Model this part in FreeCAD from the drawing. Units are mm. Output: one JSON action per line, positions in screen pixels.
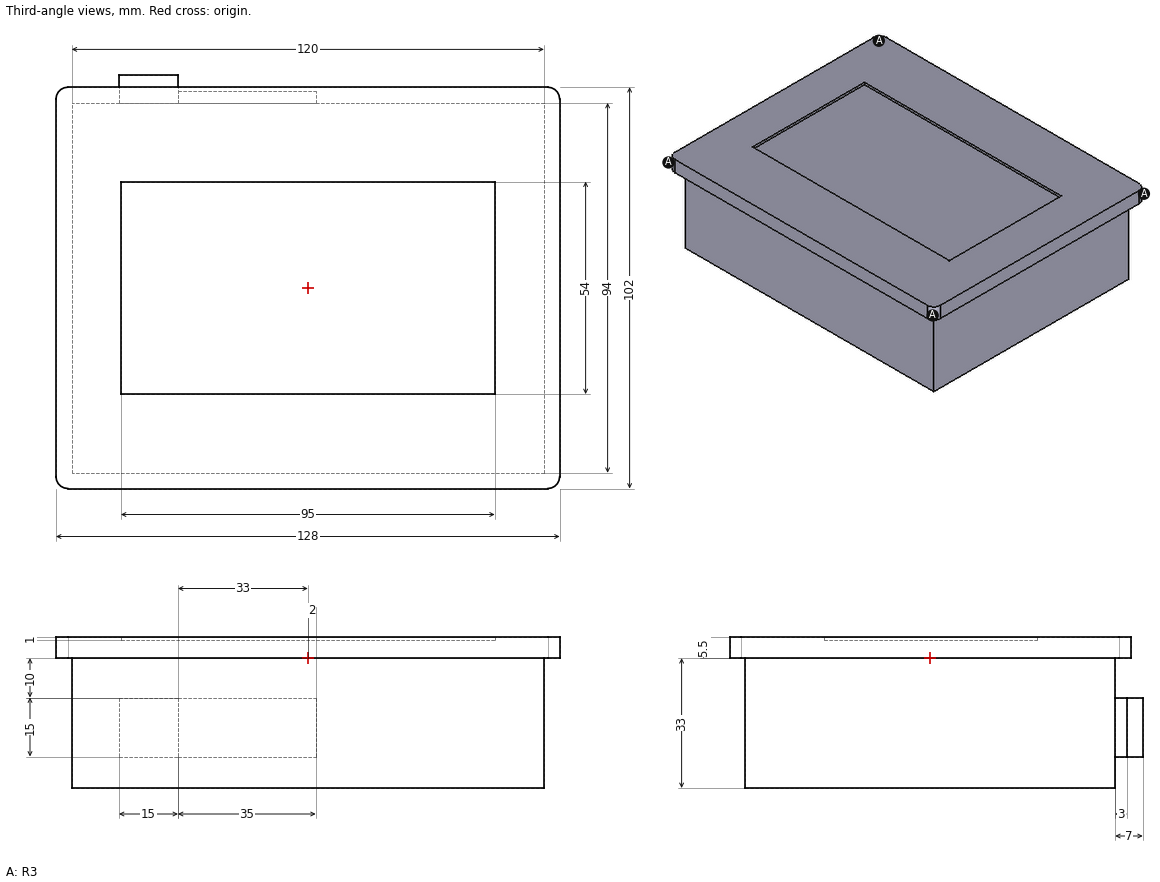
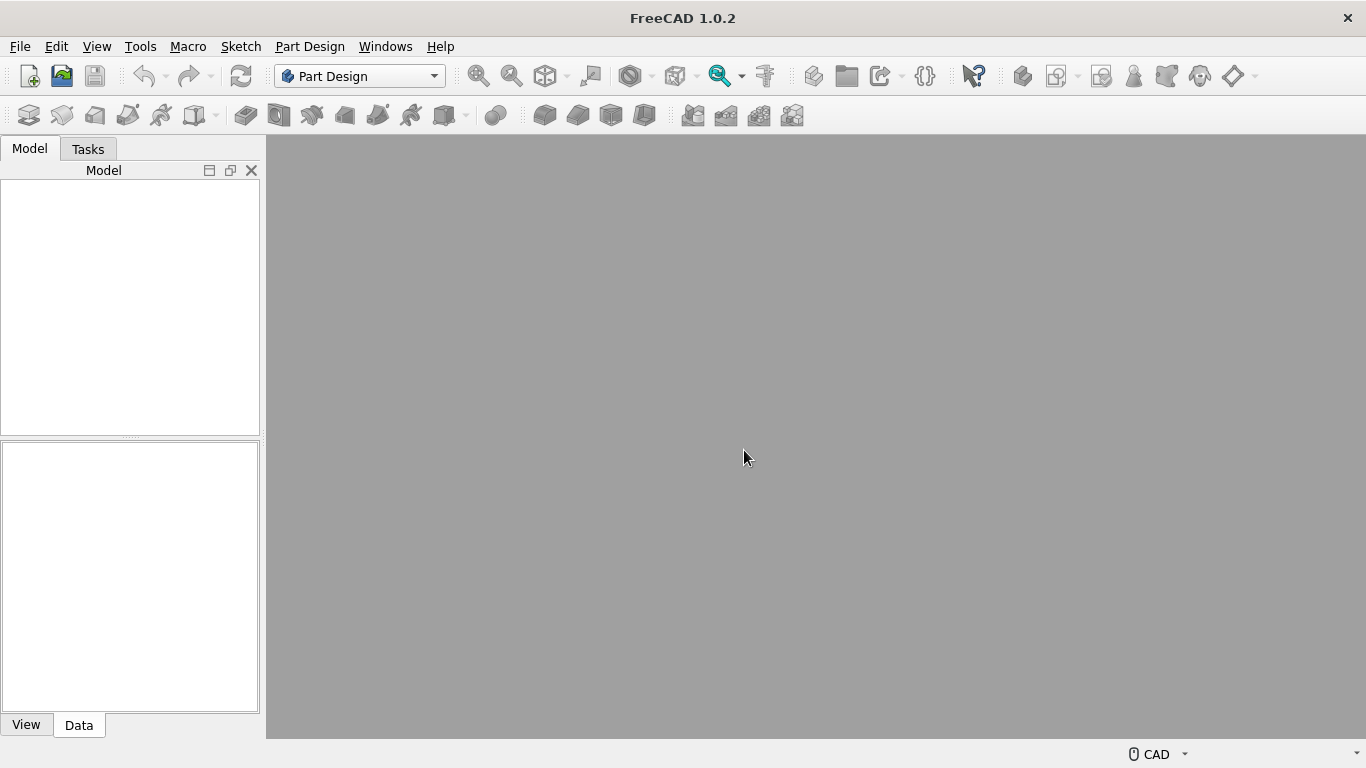
{"action": "key", "text": "ctrl+n"}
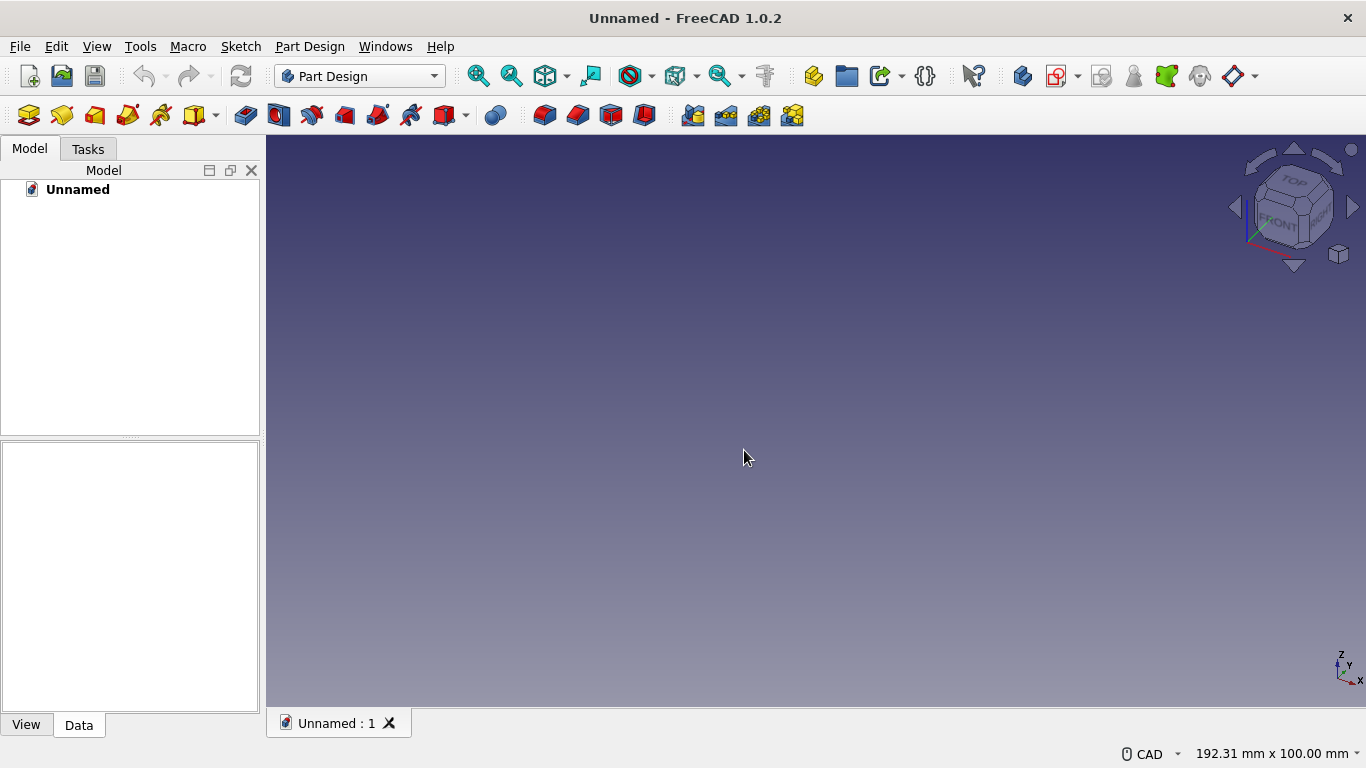
{"action": "left_click", "coordinate": [1056, 76]}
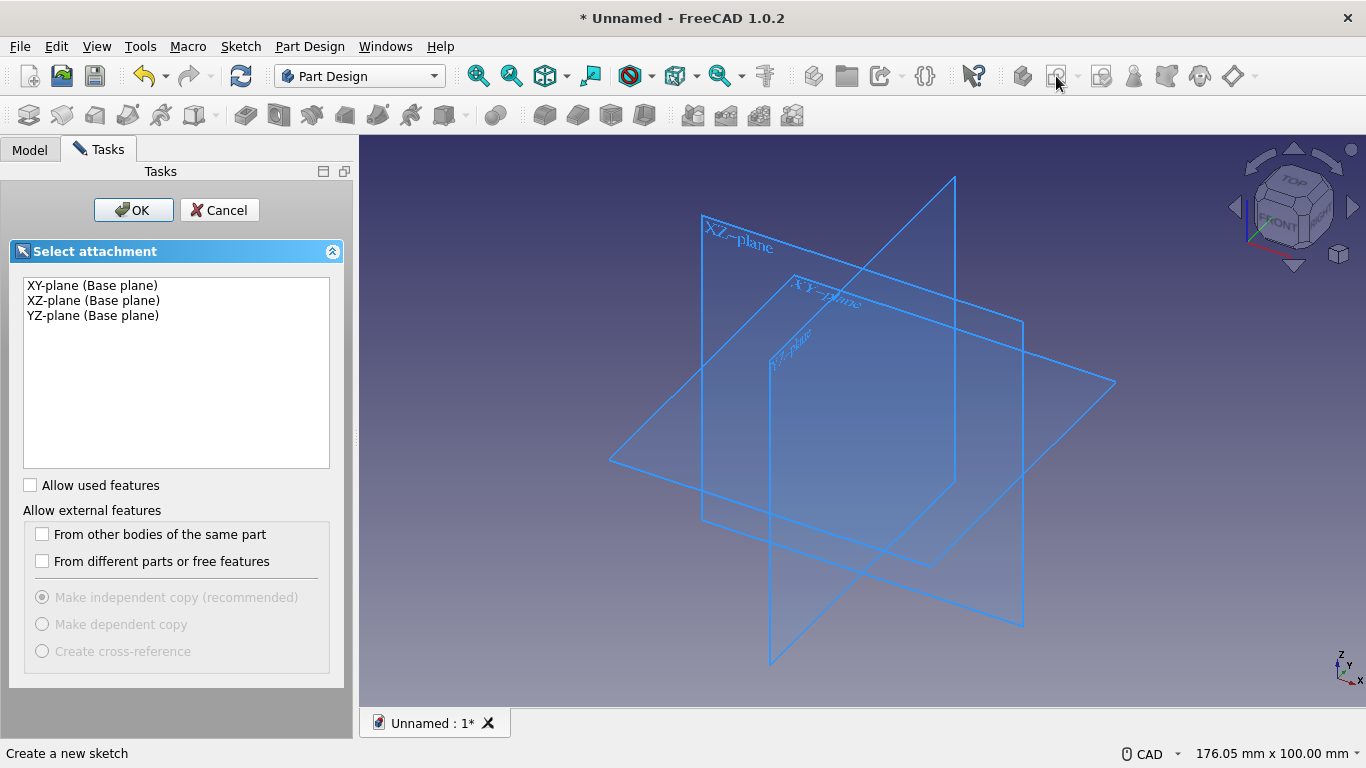
{"action": "left_click", "coordinate": [84, 286]}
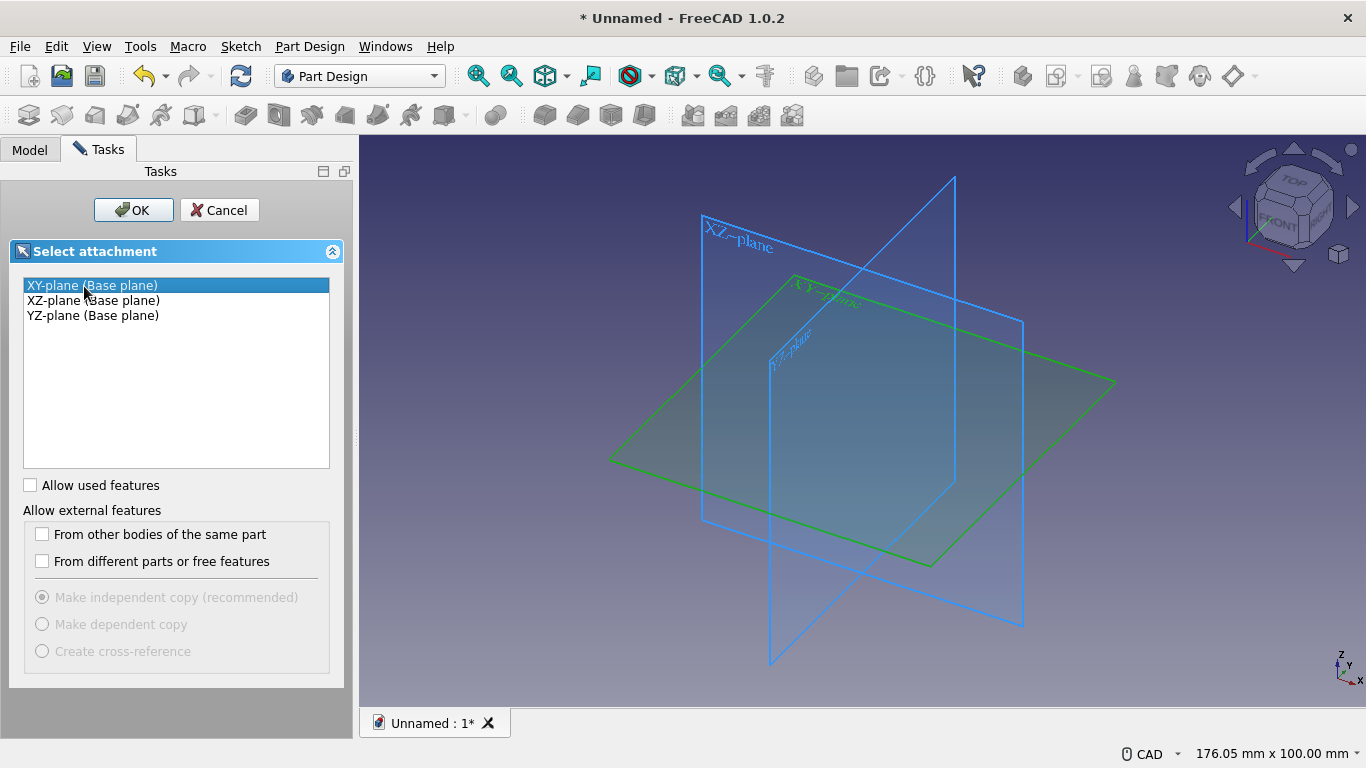
{"action": "left_click", "coordinate": [134, 210]}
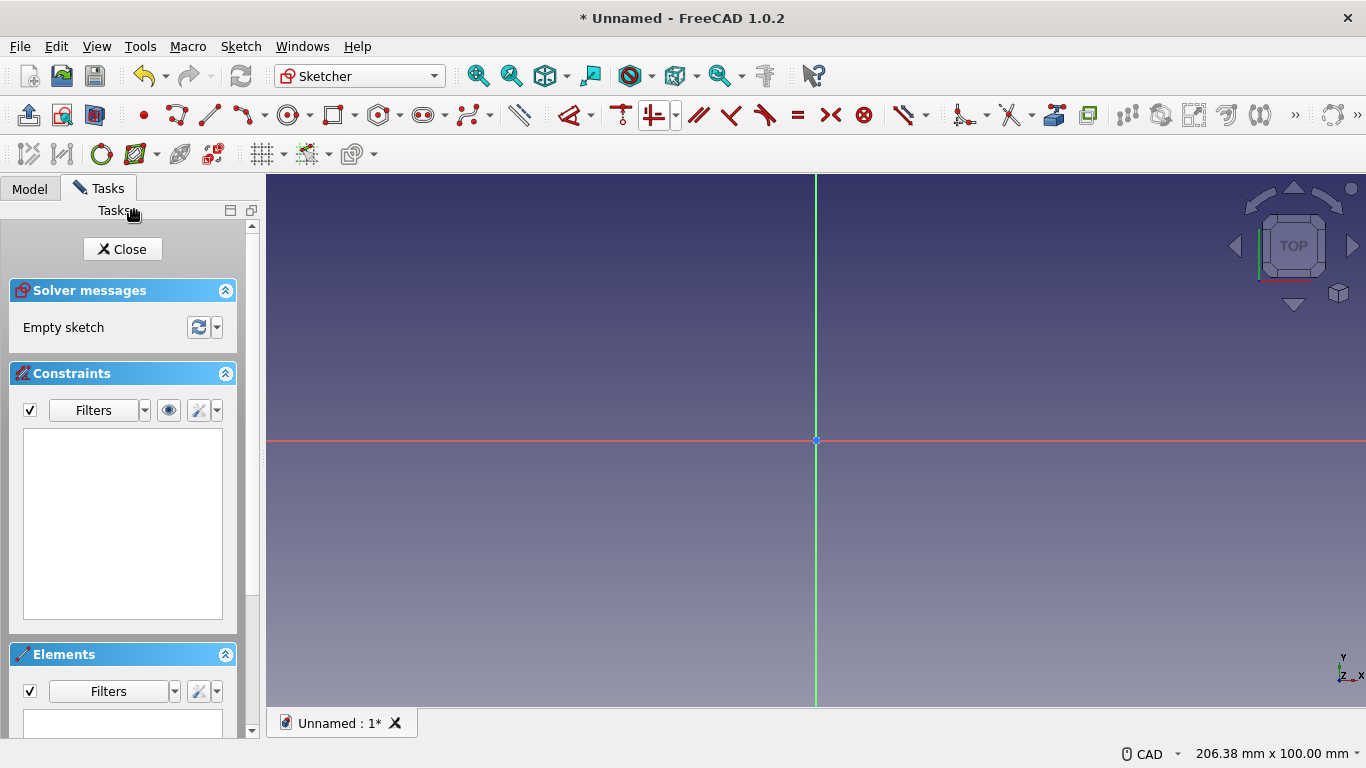
{"action": "scroll", "coordinate": [608, 440], "scroll_direction": "down", "scroll_amount": 2}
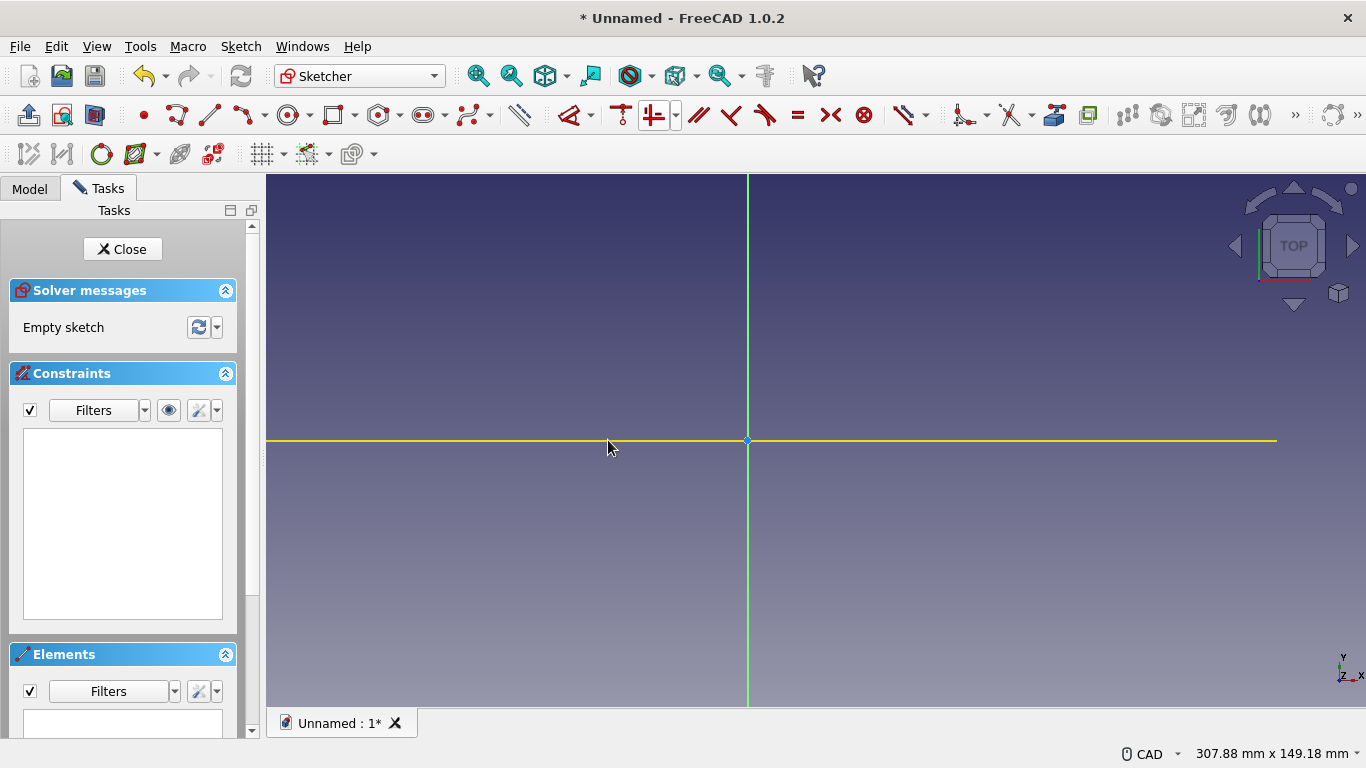
{"action": "left_click", "coordinate": [354, 116]}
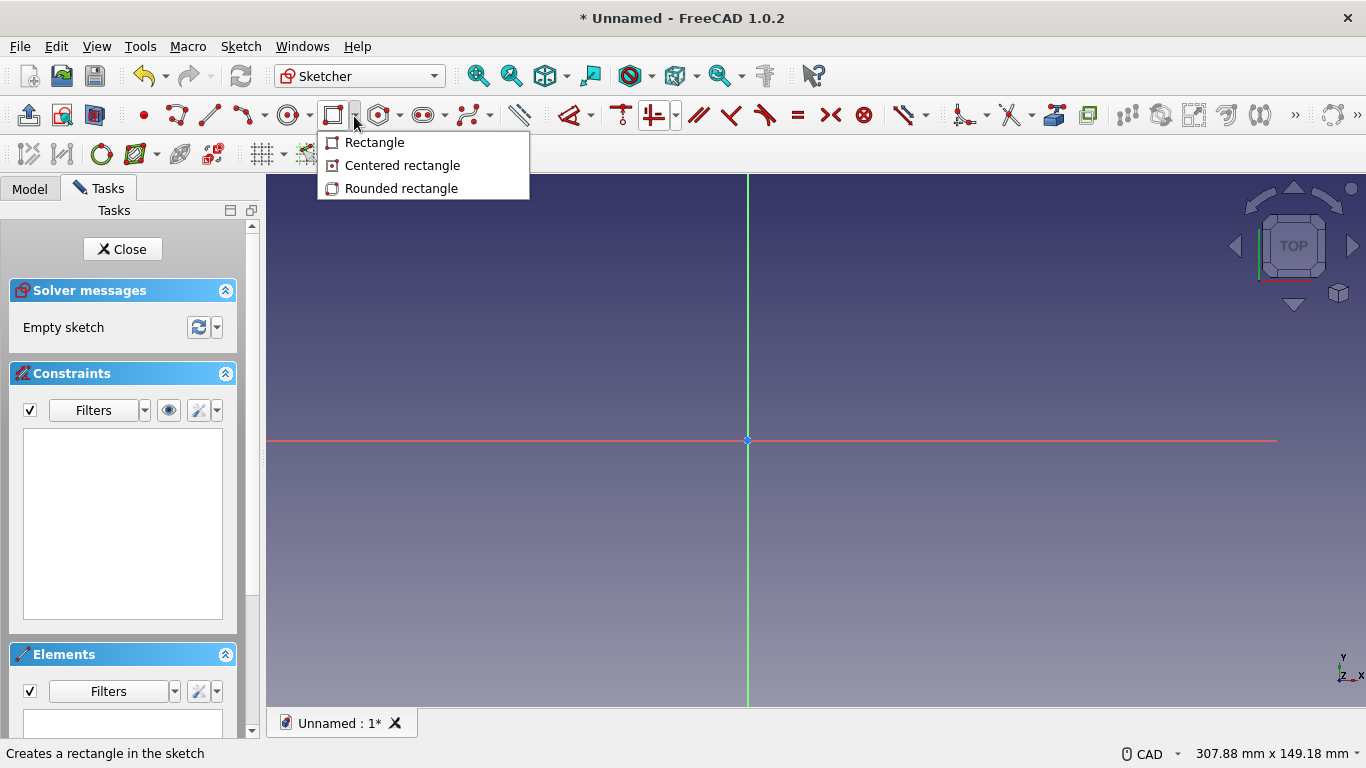
{"action": "left_click", "coordinate": [424, 166]}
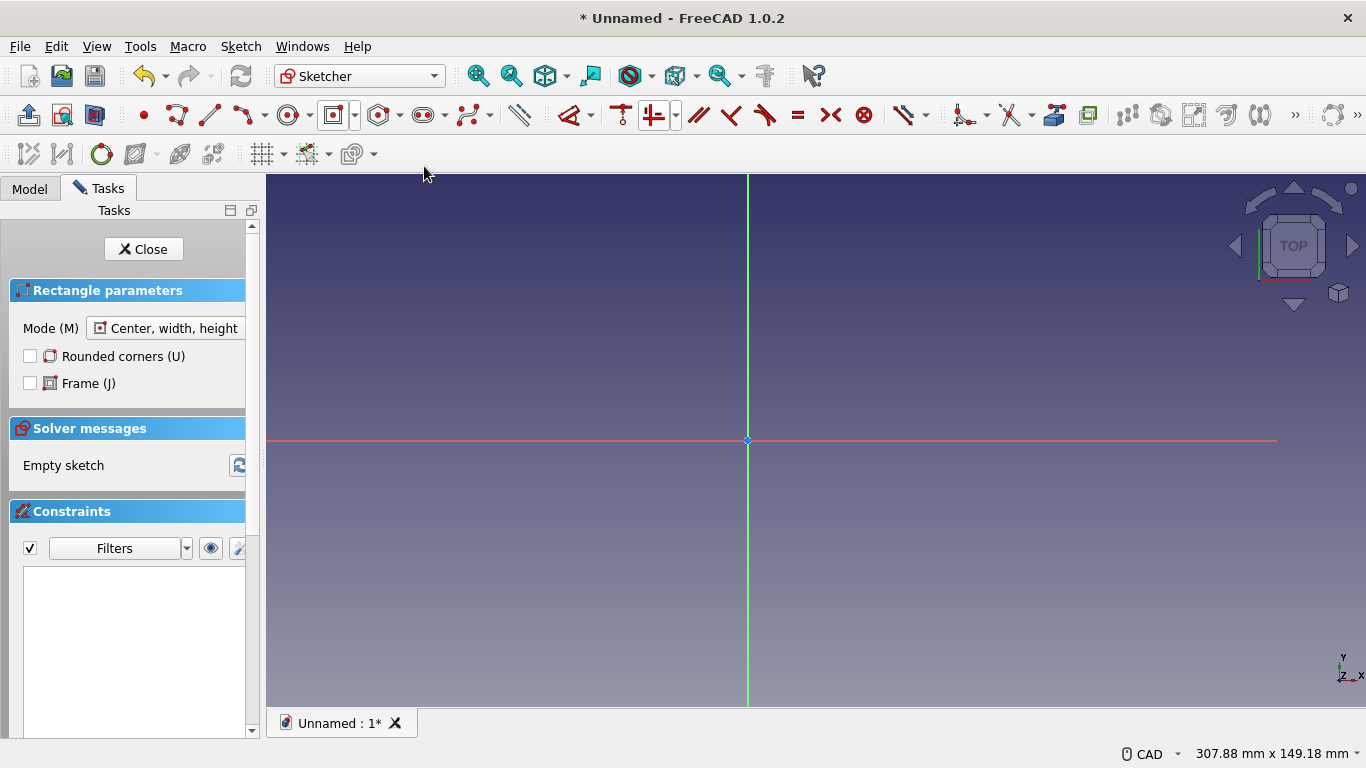
{"action": "left_click", "coordinate": [748, 440]}
{"action": "mouse_move", "coordinate": [976, 258]}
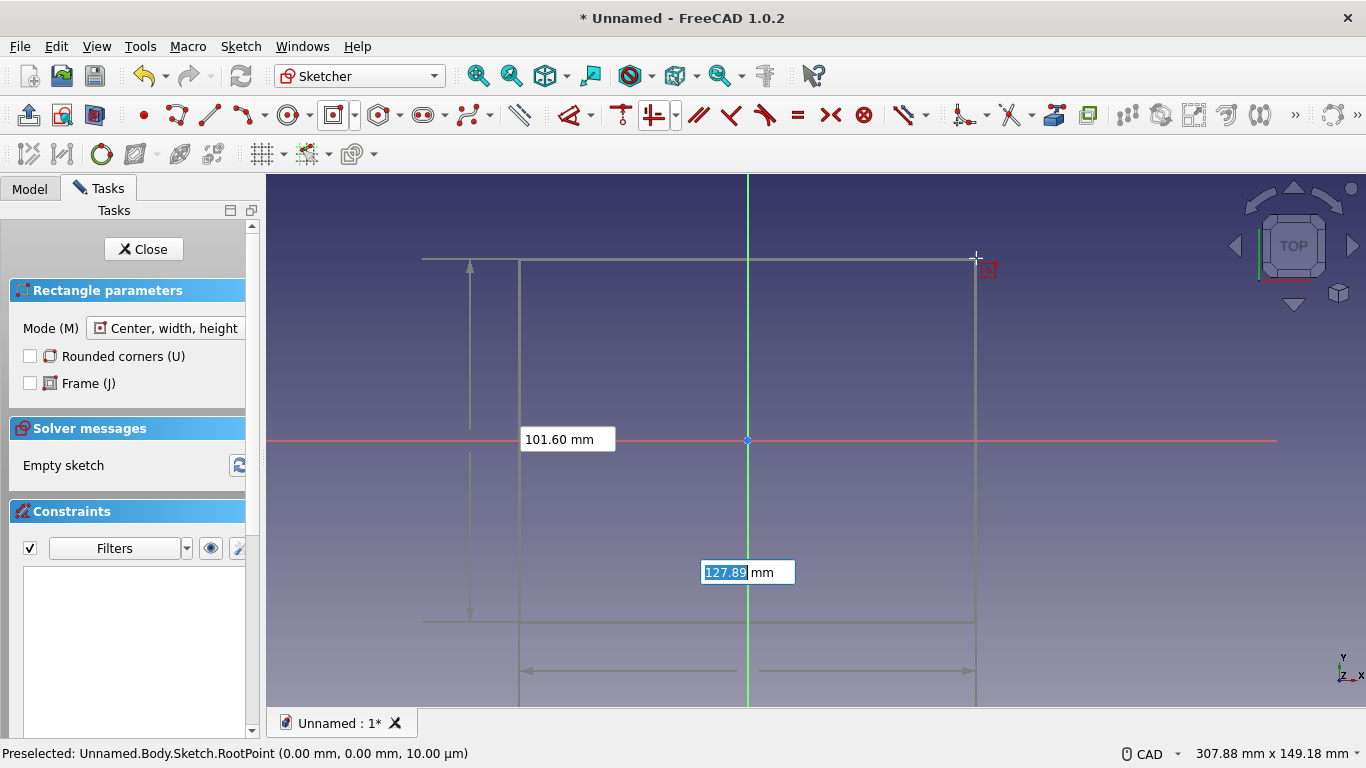
{"action": "type", "text": "128"}
{"action": "key", "text": "Tab"}
{"action": "type", "text": "102"}
{"action": "key", "text": "Return"}
{"action": "key", "text": "Escape"}